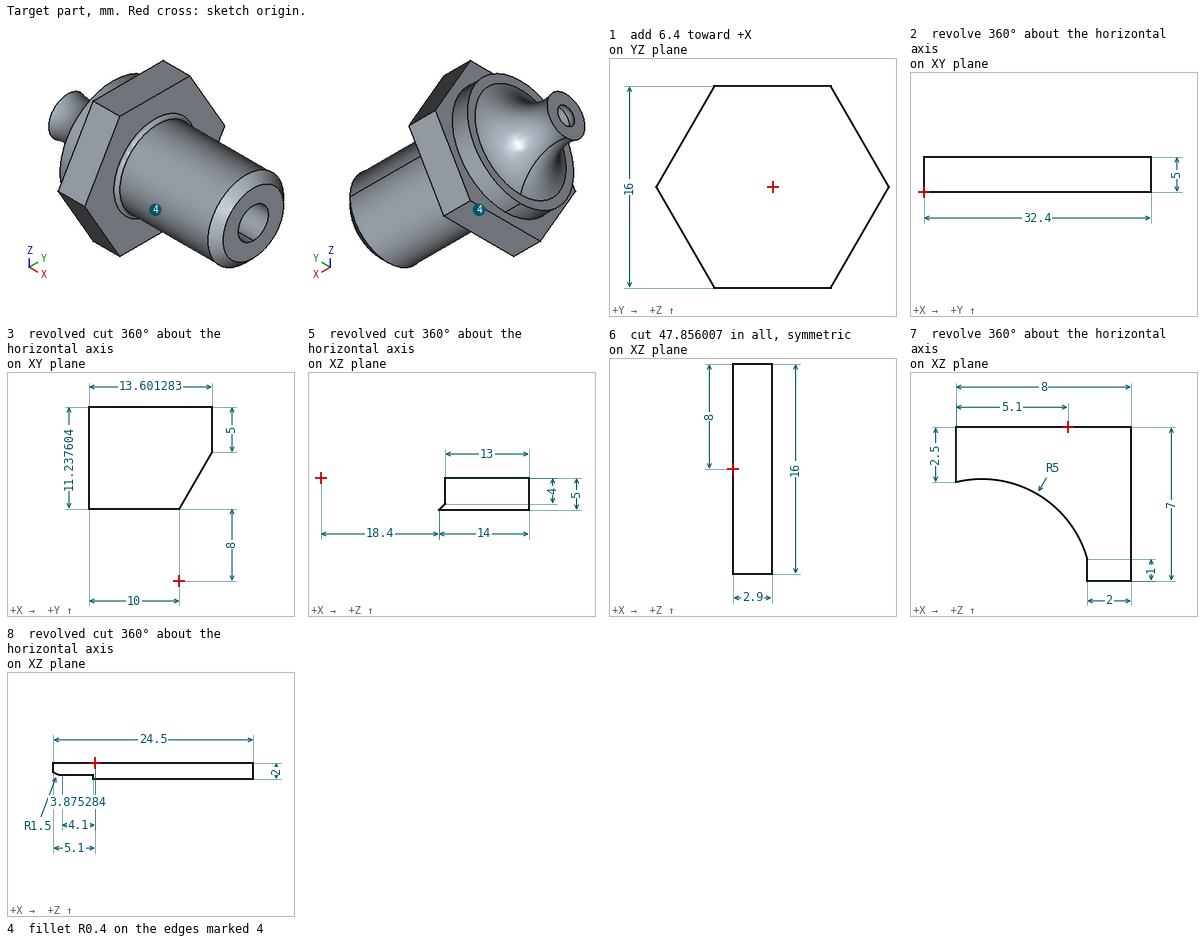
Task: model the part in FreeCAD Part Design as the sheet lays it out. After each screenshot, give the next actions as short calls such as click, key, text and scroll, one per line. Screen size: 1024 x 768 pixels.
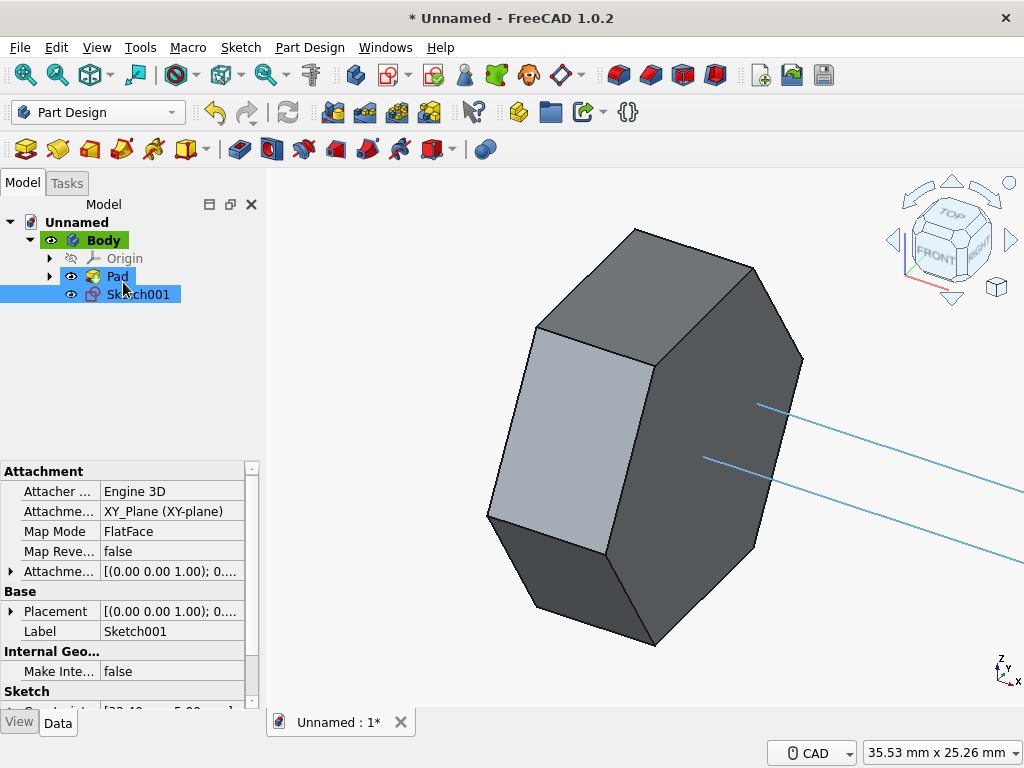
click(58, 150)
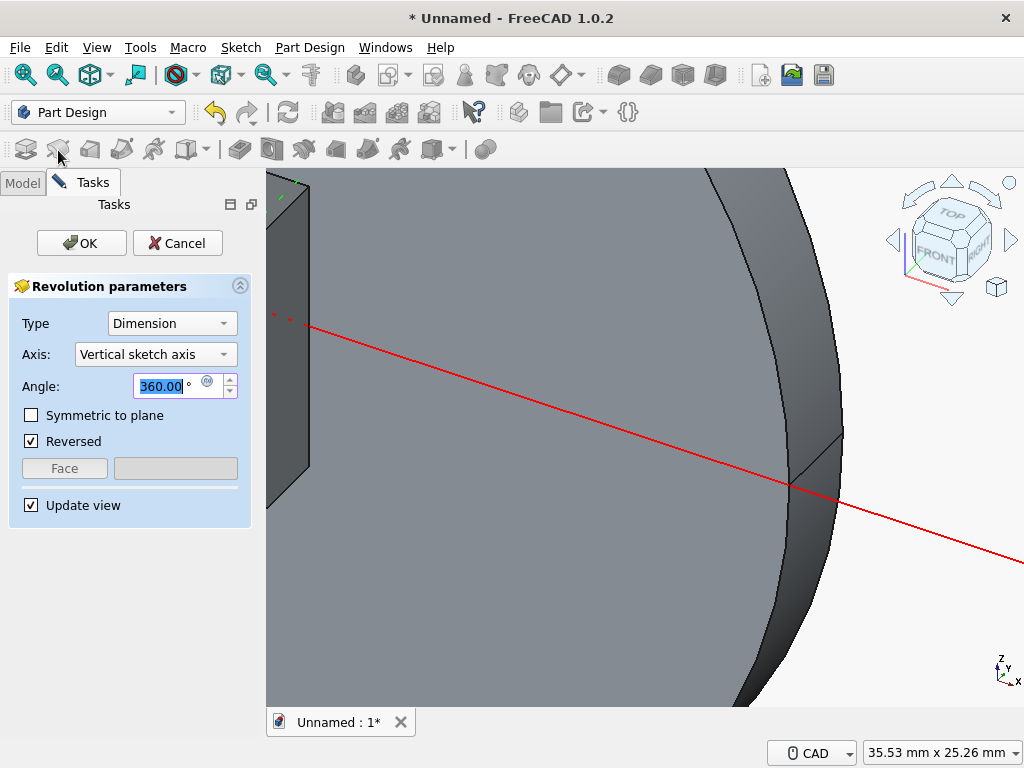
click(156, 354)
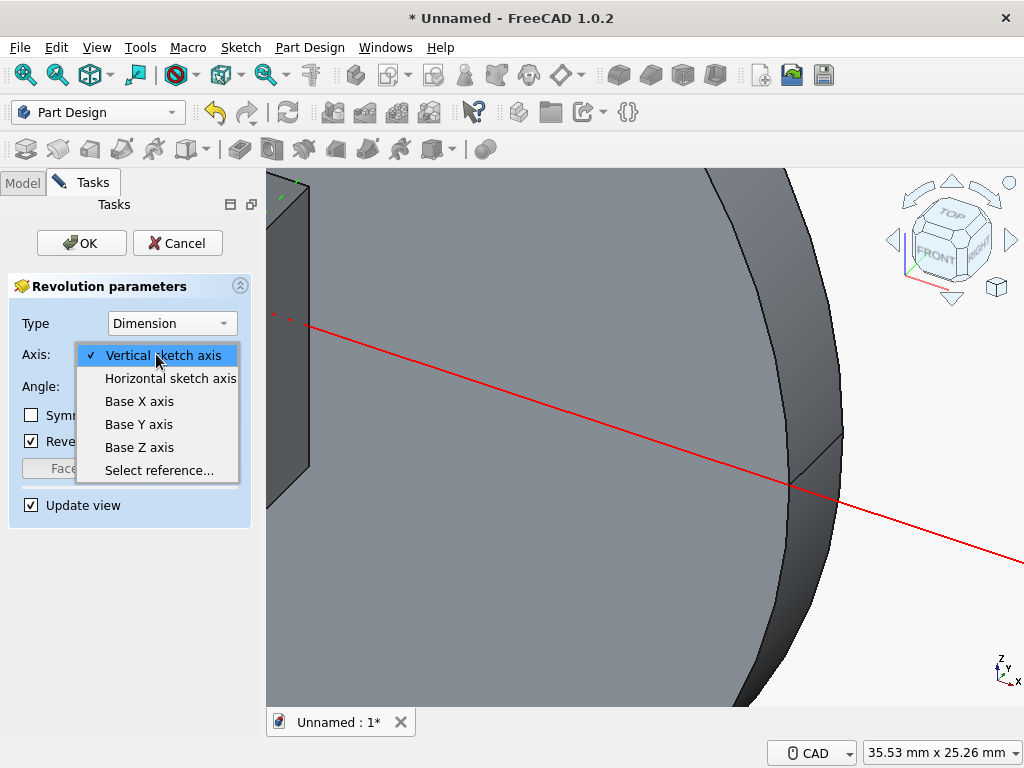
click(156, 378)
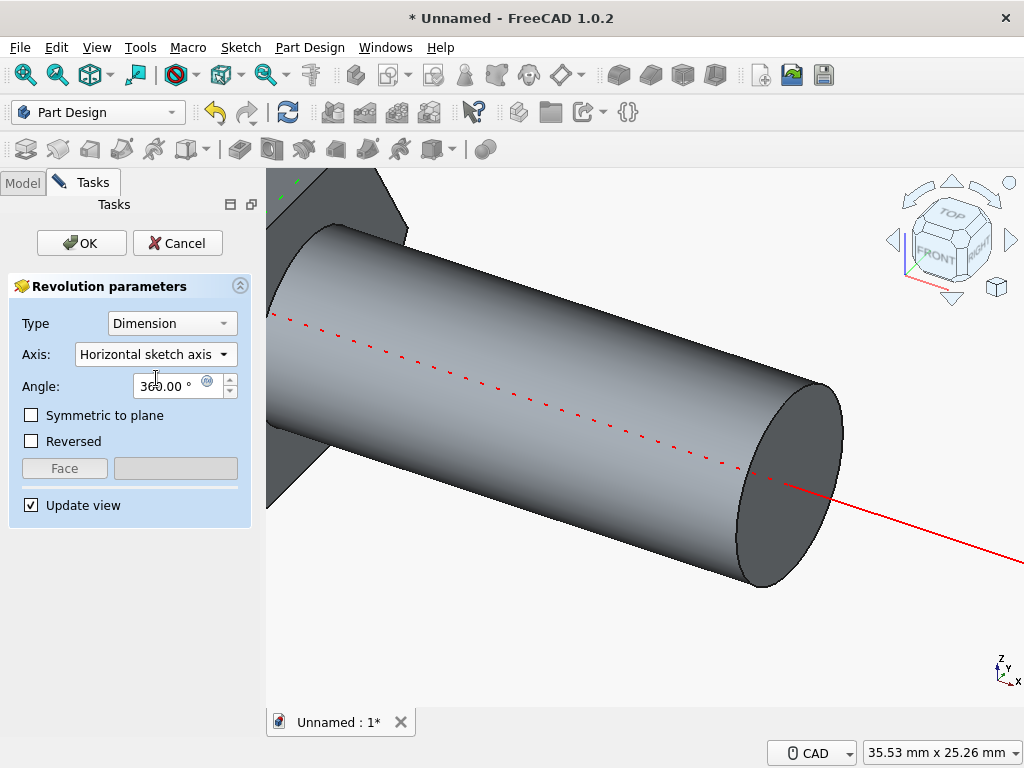
click(82, 243)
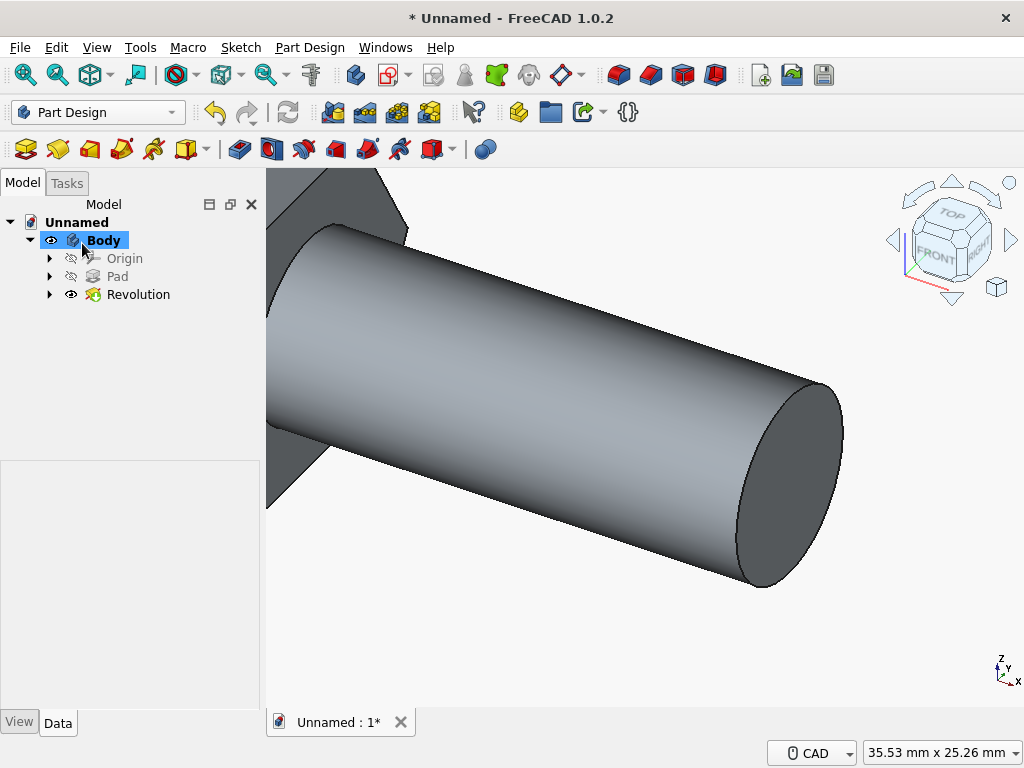
click(26, 76)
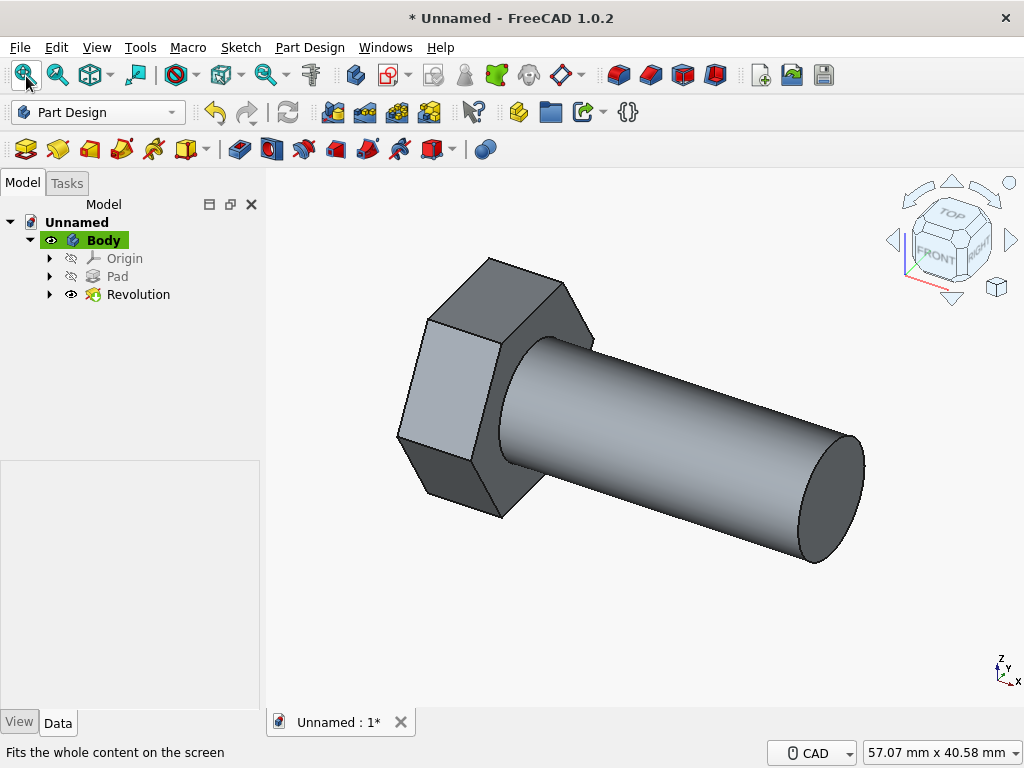
click(388, 76)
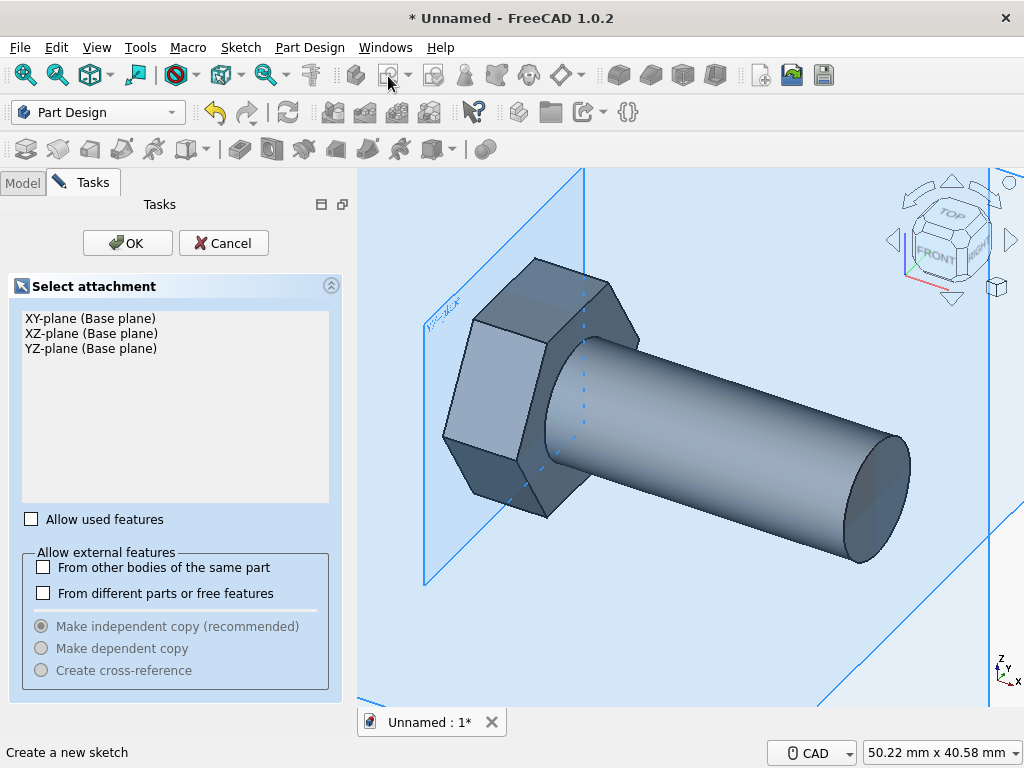
click(82, 318)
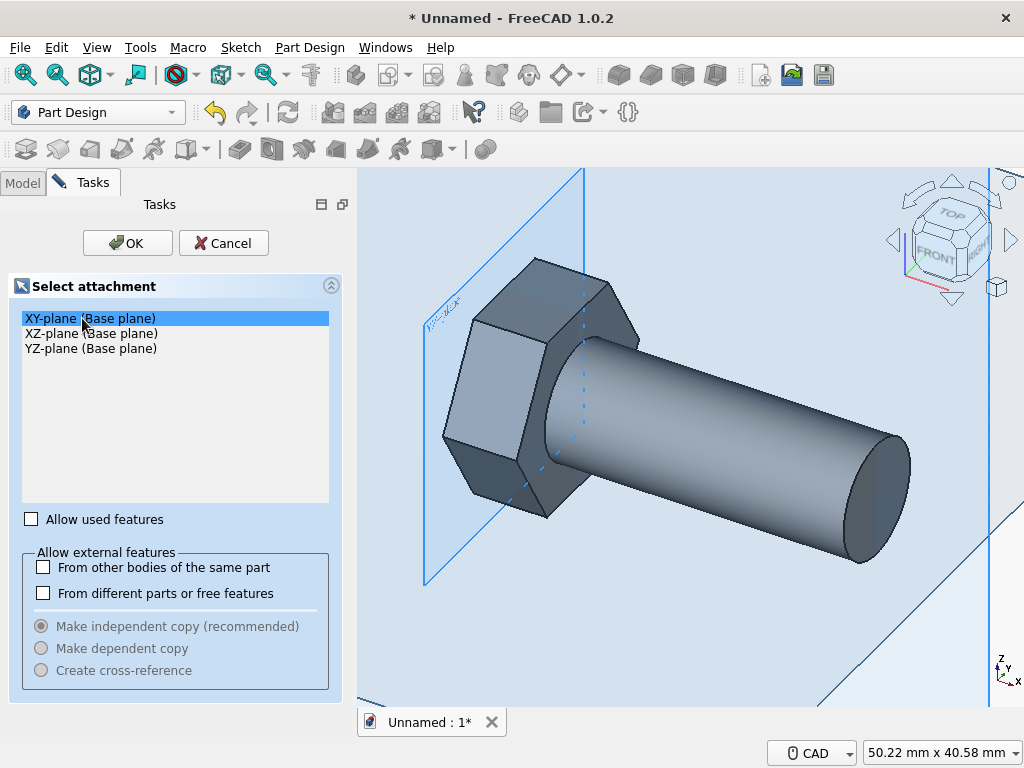
click(128, 243)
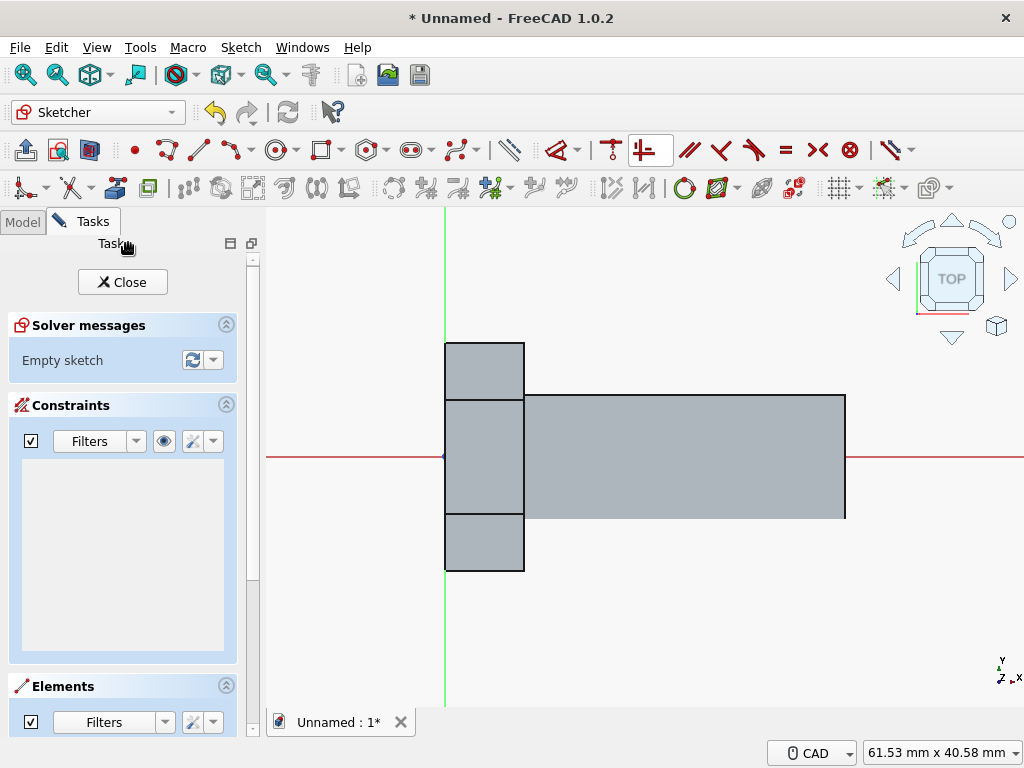
click(90, 150)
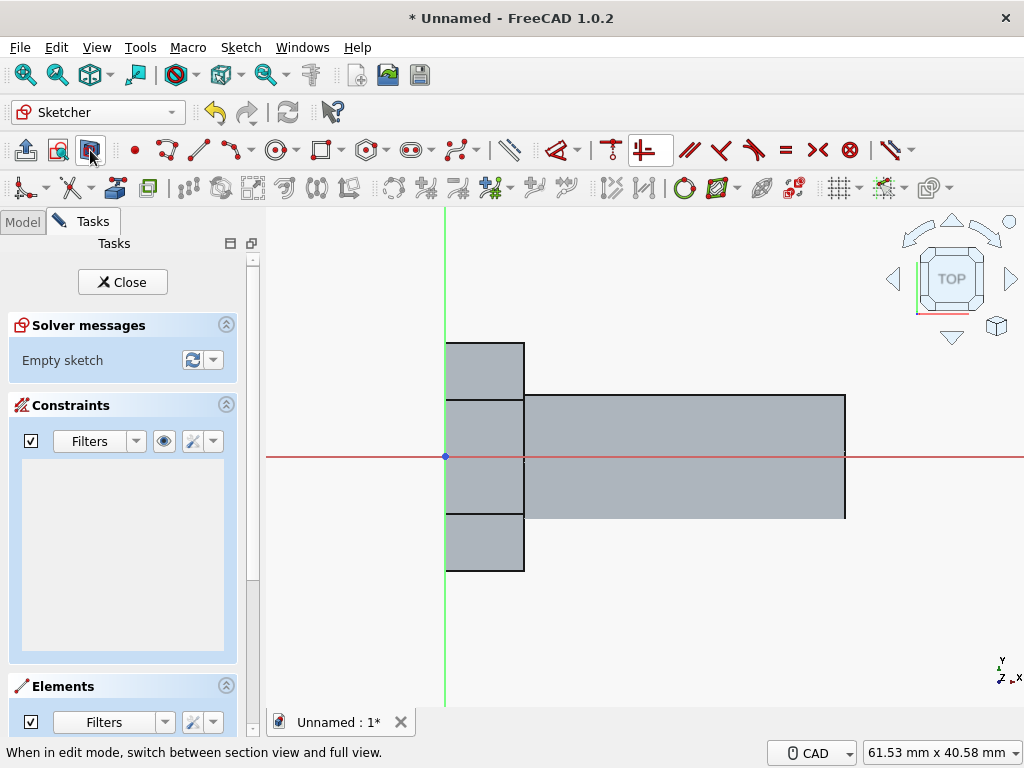
scroll(859, 679, down, 1)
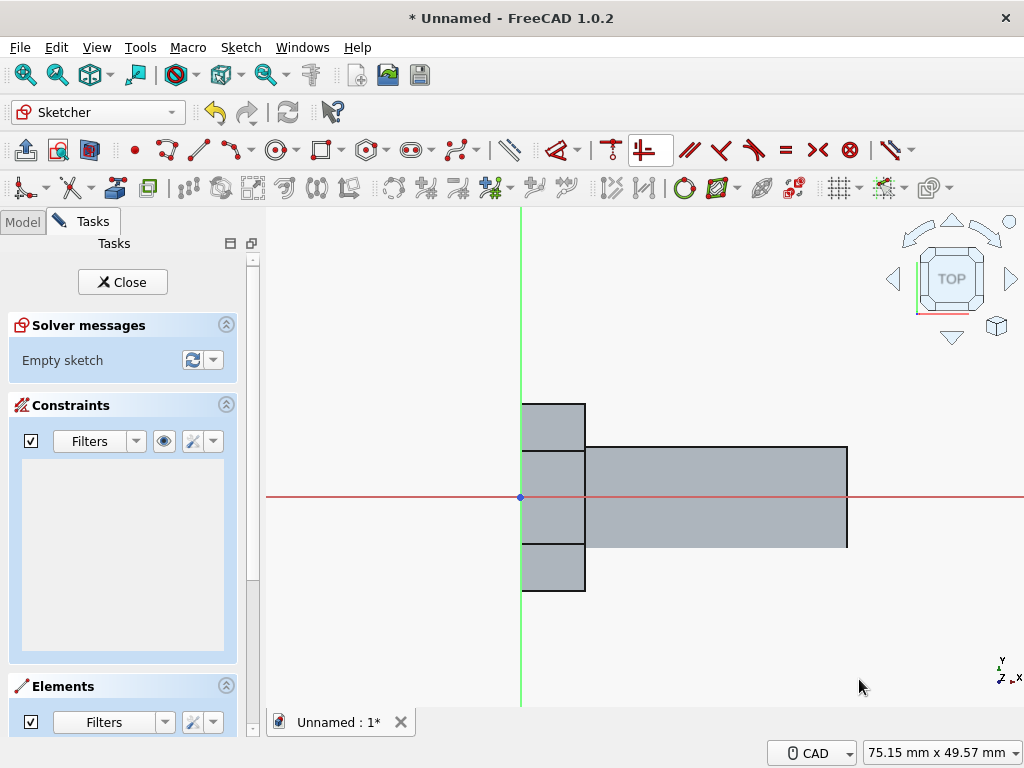
scroll(309, 285, up, 2)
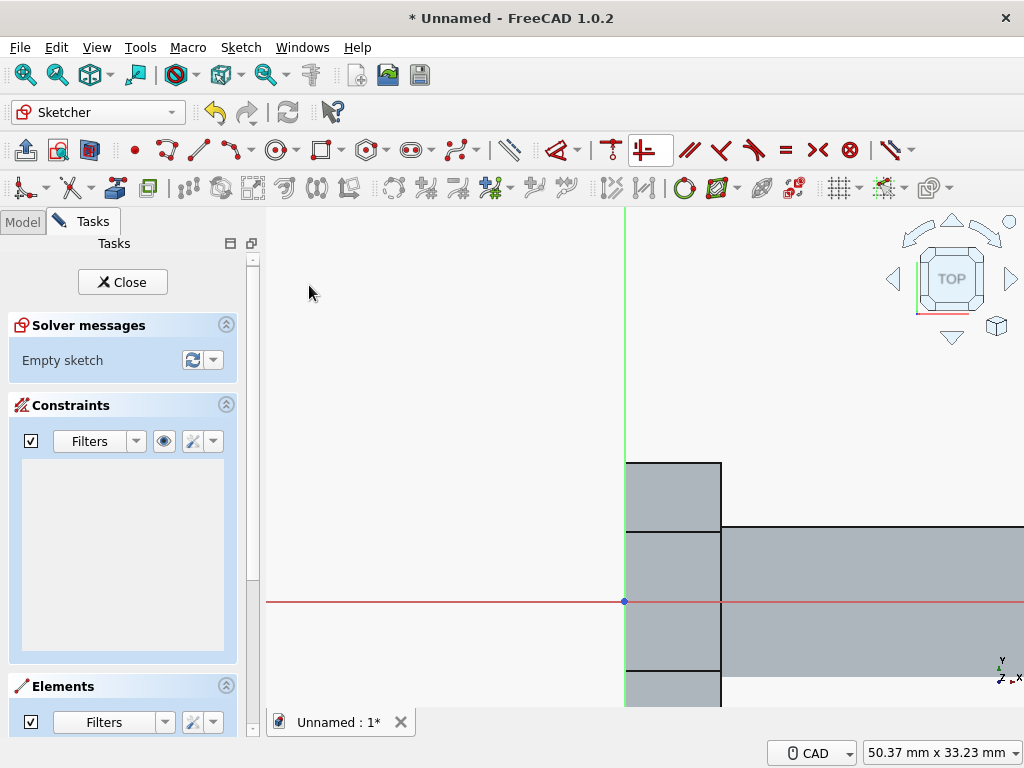
click(168, 150)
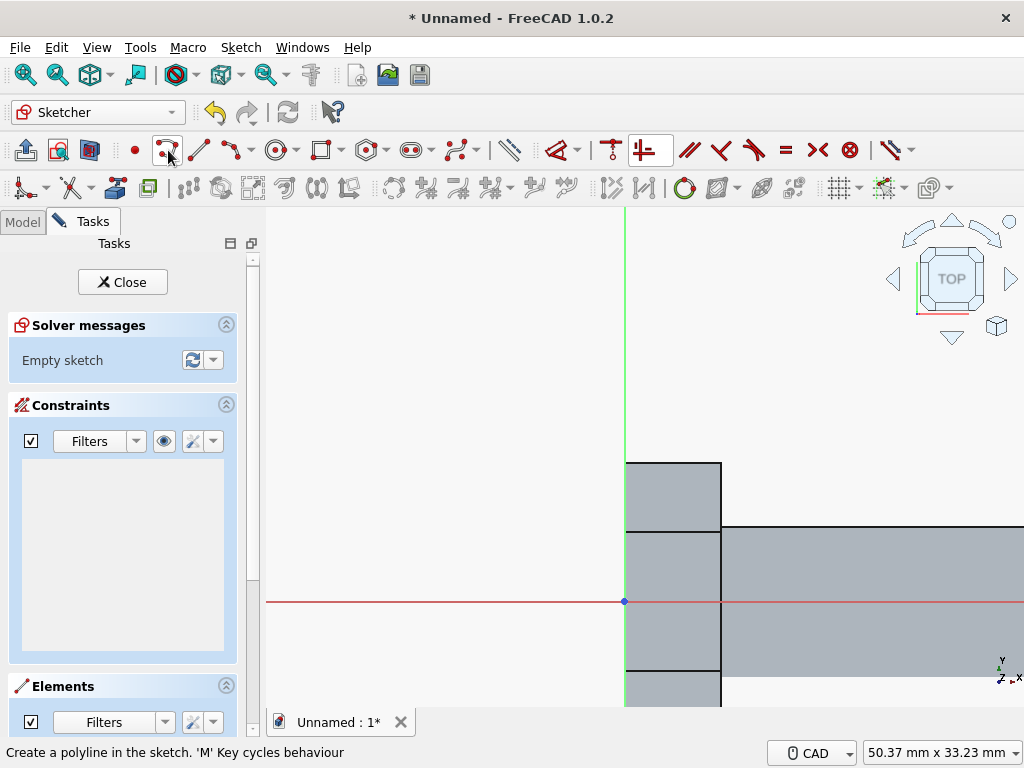
click(625, 481)
click(679, 388)
click(679, 312)
click(474, 312)
click(474, 481)
click(625, 482)
key(Escape)
key(Escape)